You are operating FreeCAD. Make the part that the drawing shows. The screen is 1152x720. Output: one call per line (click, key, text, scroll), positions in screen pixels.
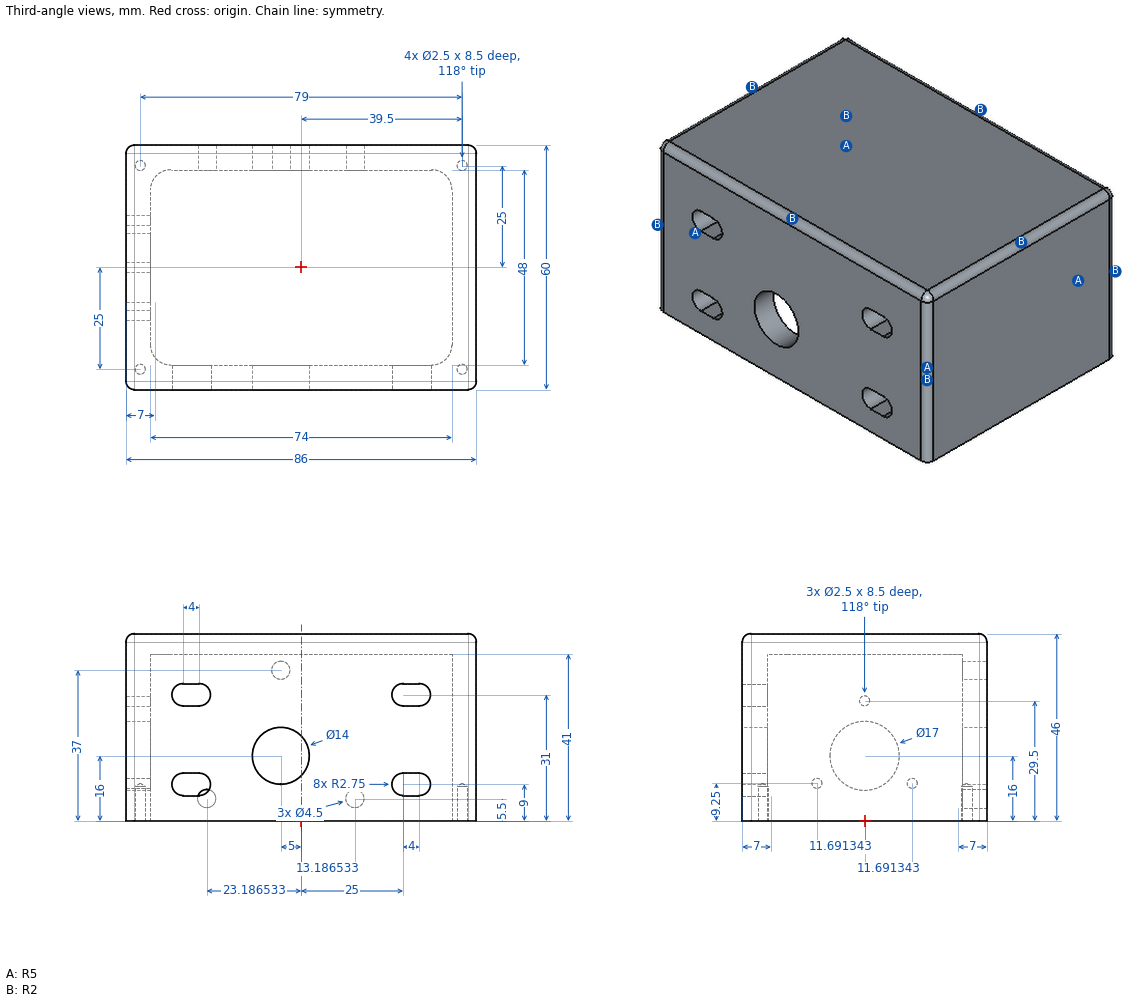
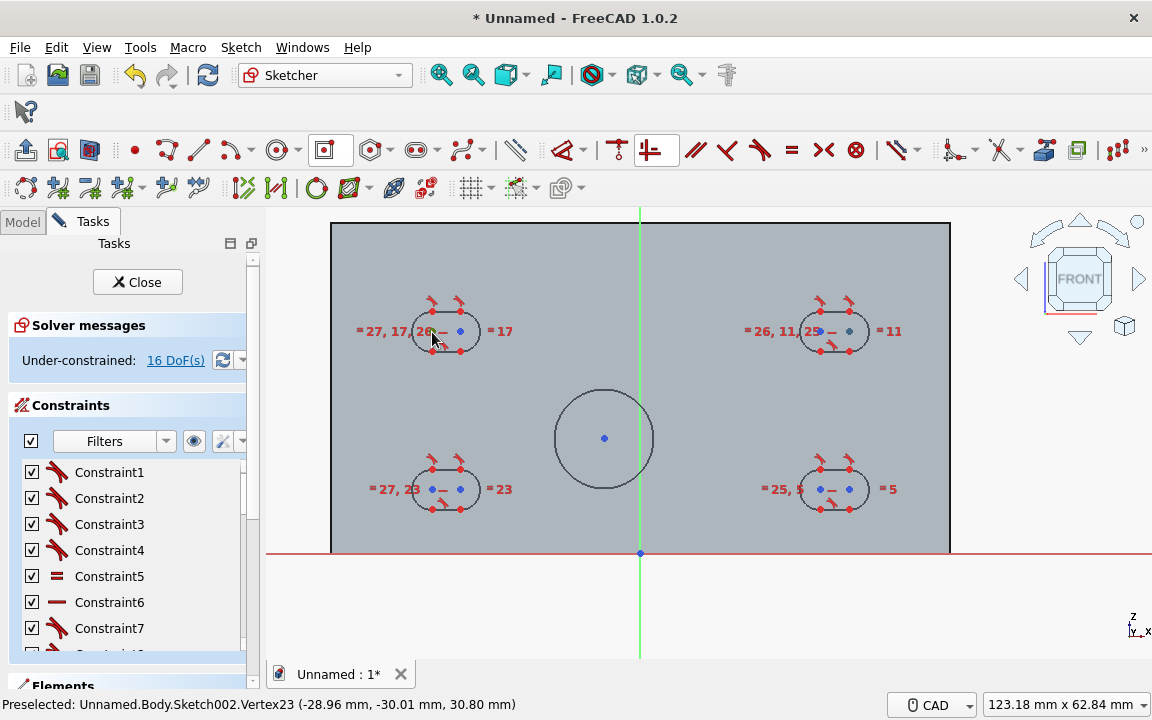
click(640, 603)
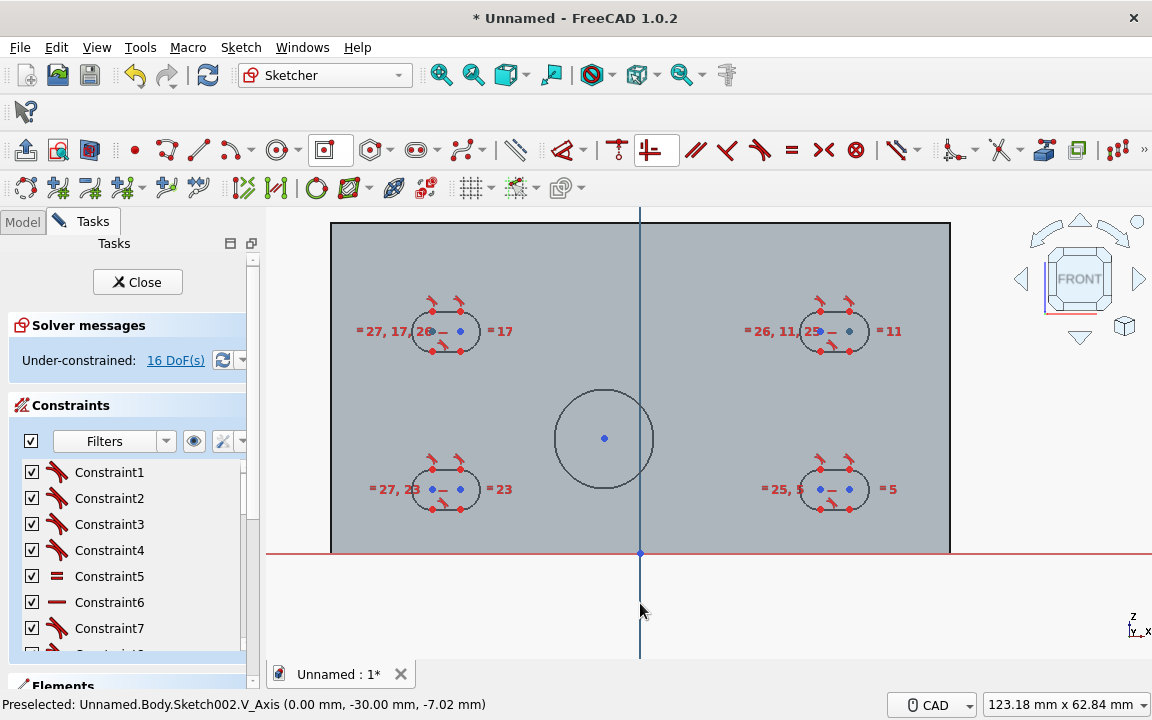
key(s)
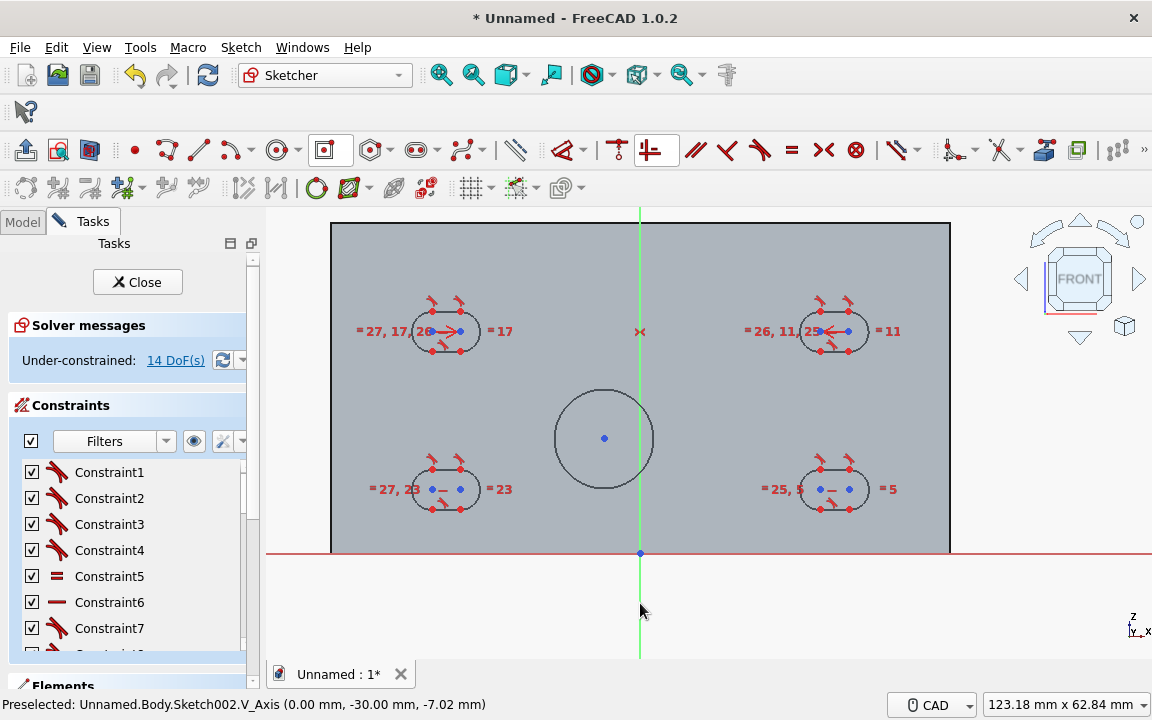
click(849, 490)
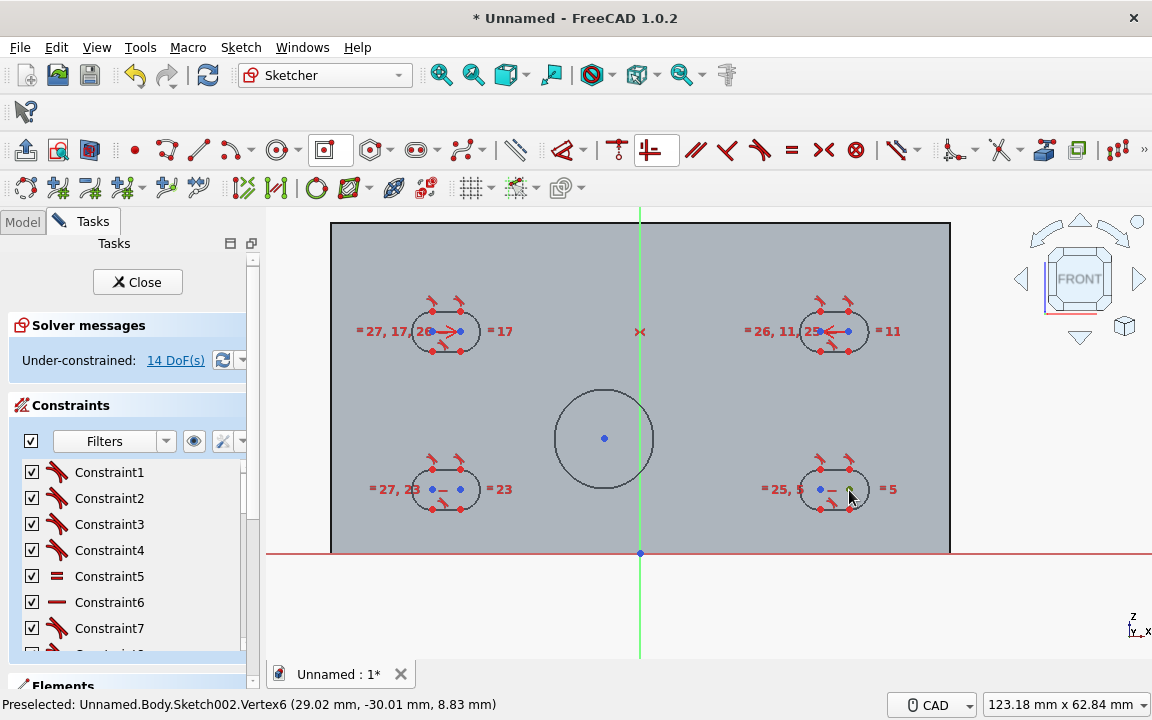
click(432, 490)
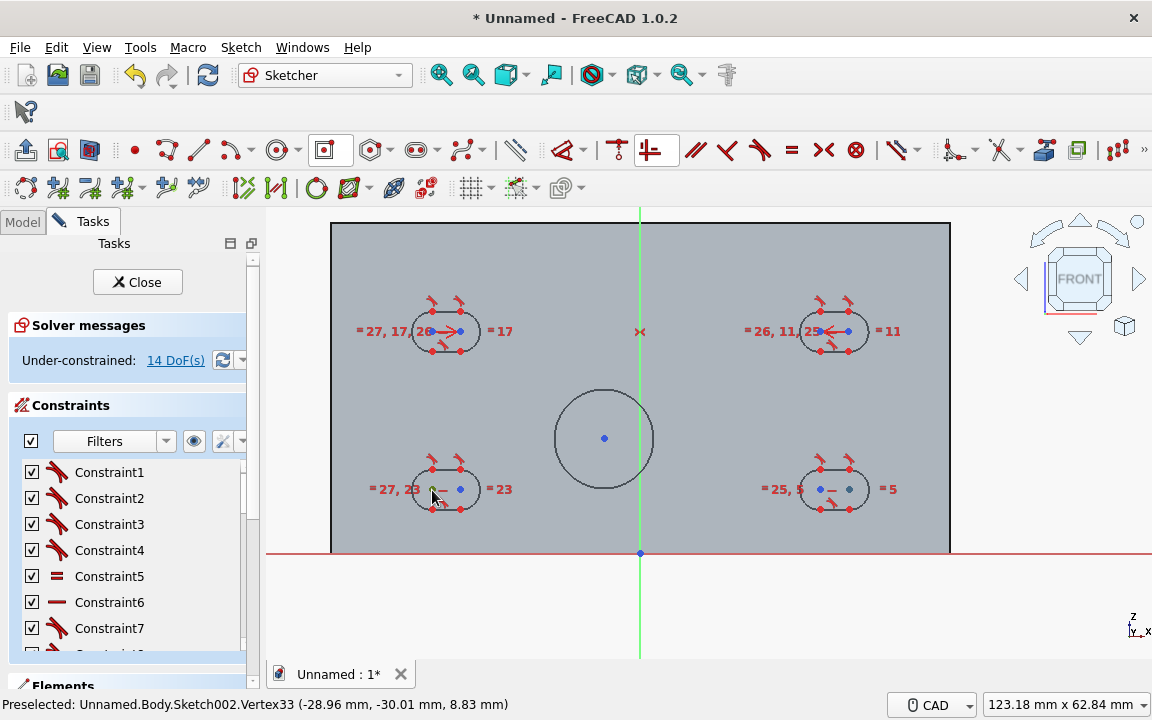
click(640, 603)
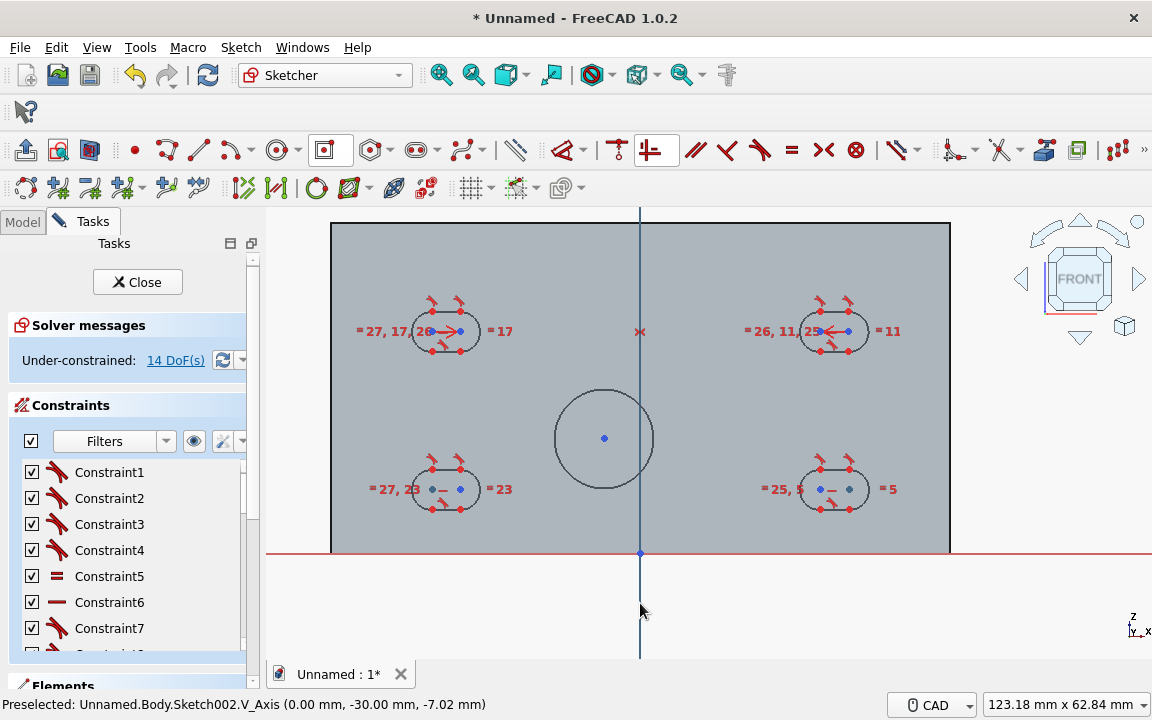
key(s)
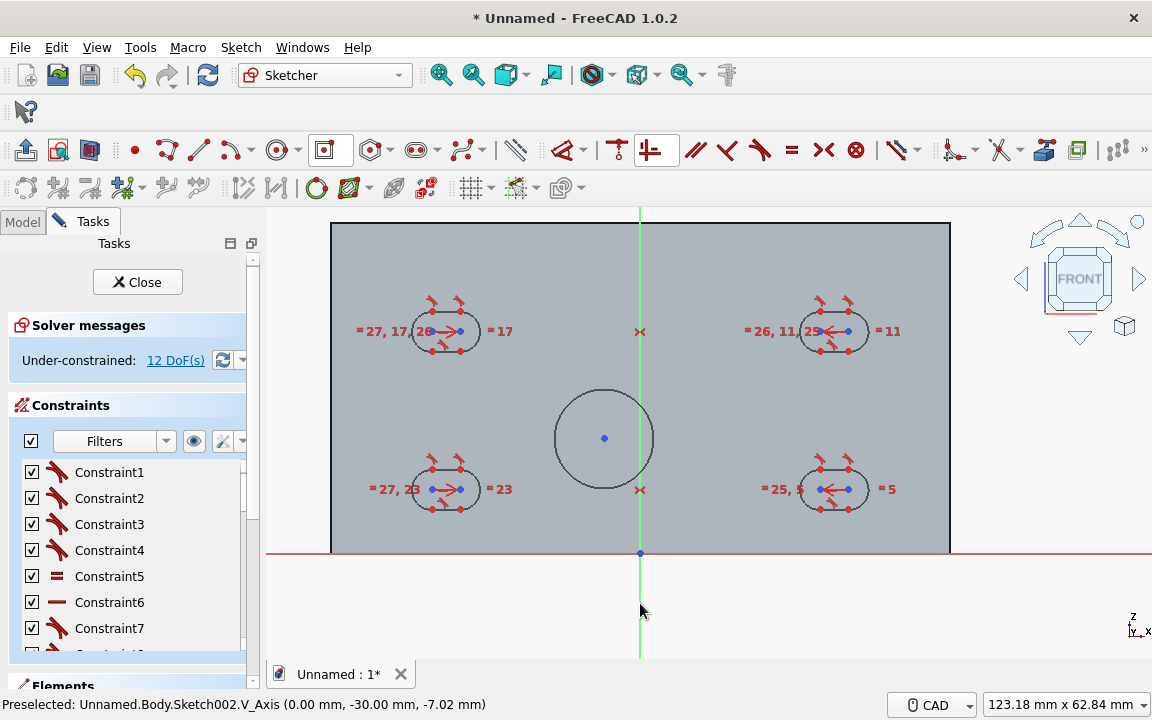
click(562, 150)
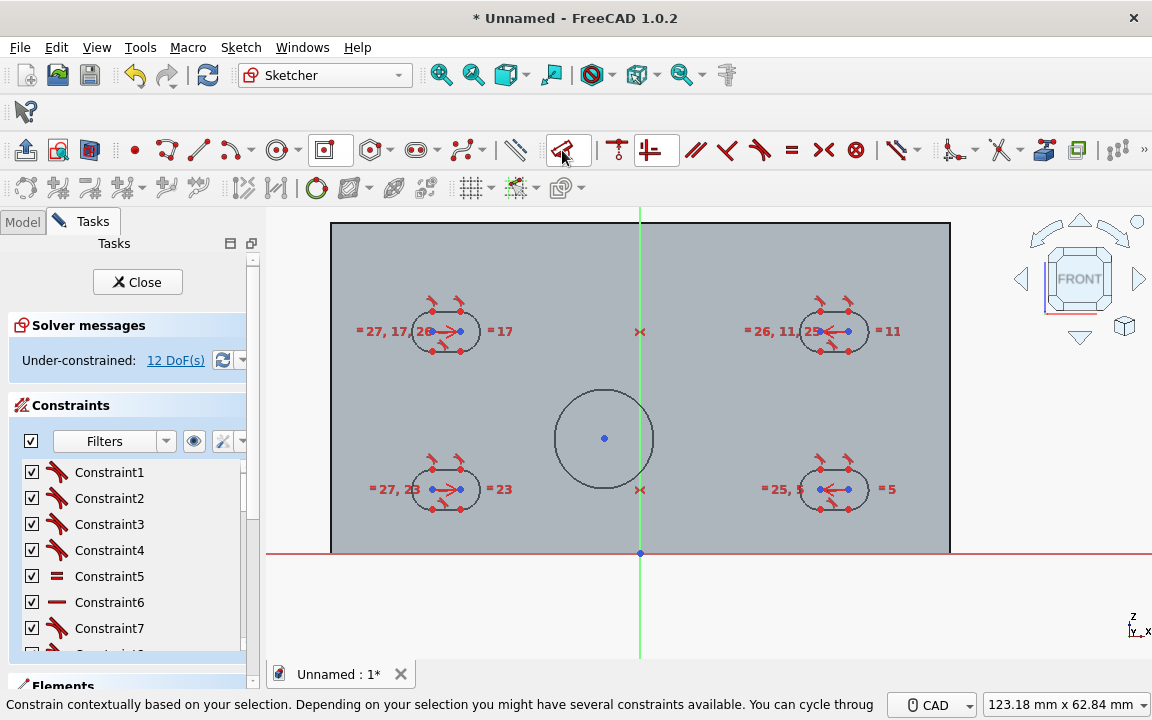
scroll(804, 478, up, 4)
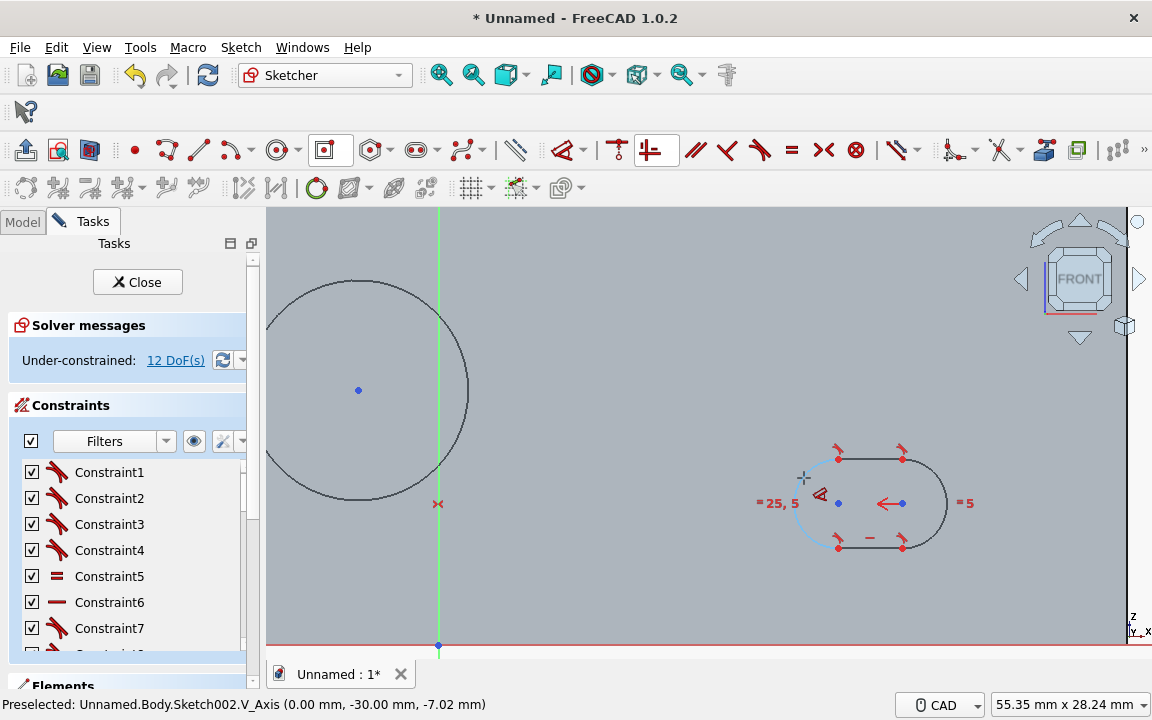
click(803, 478)
click(777, 459)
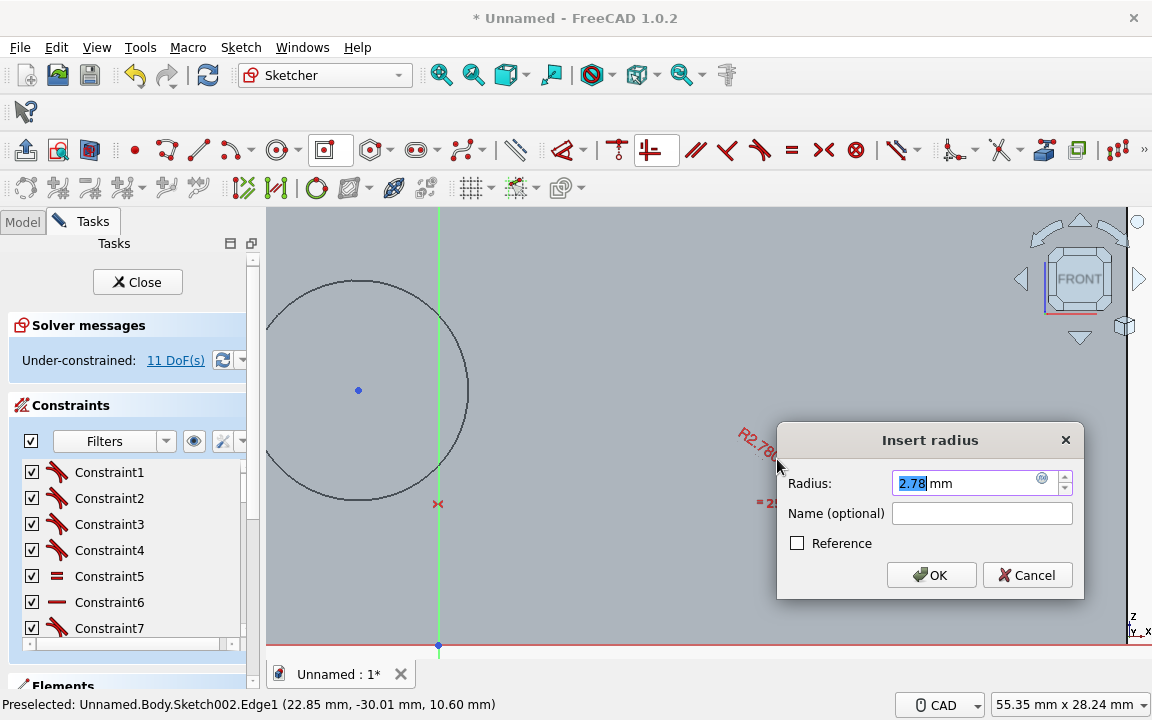
text(2.75)
key(Return)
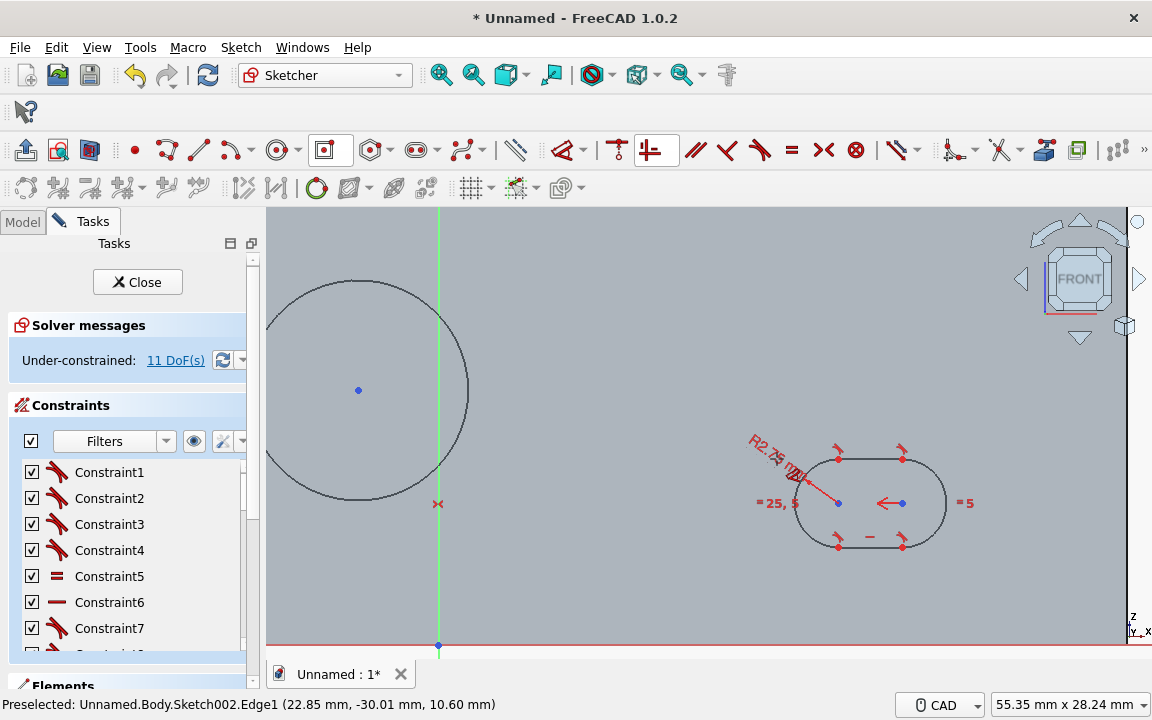
click(436, 312)
click(459, 289)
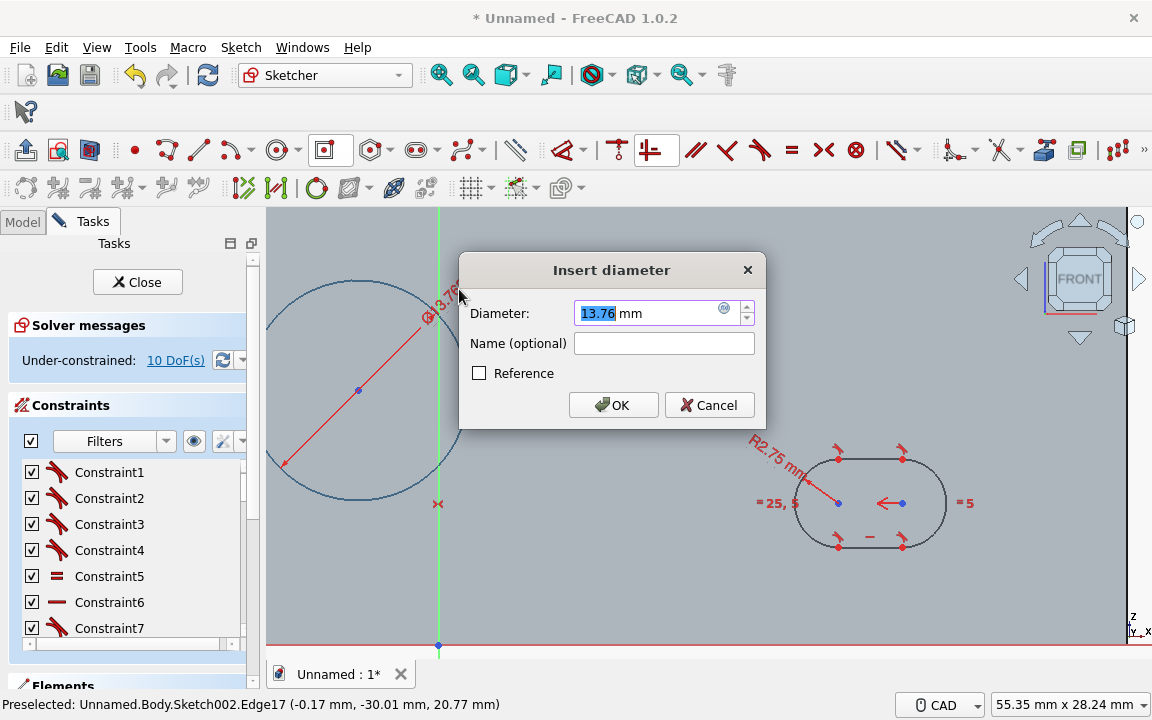
text(14)
key(Return)